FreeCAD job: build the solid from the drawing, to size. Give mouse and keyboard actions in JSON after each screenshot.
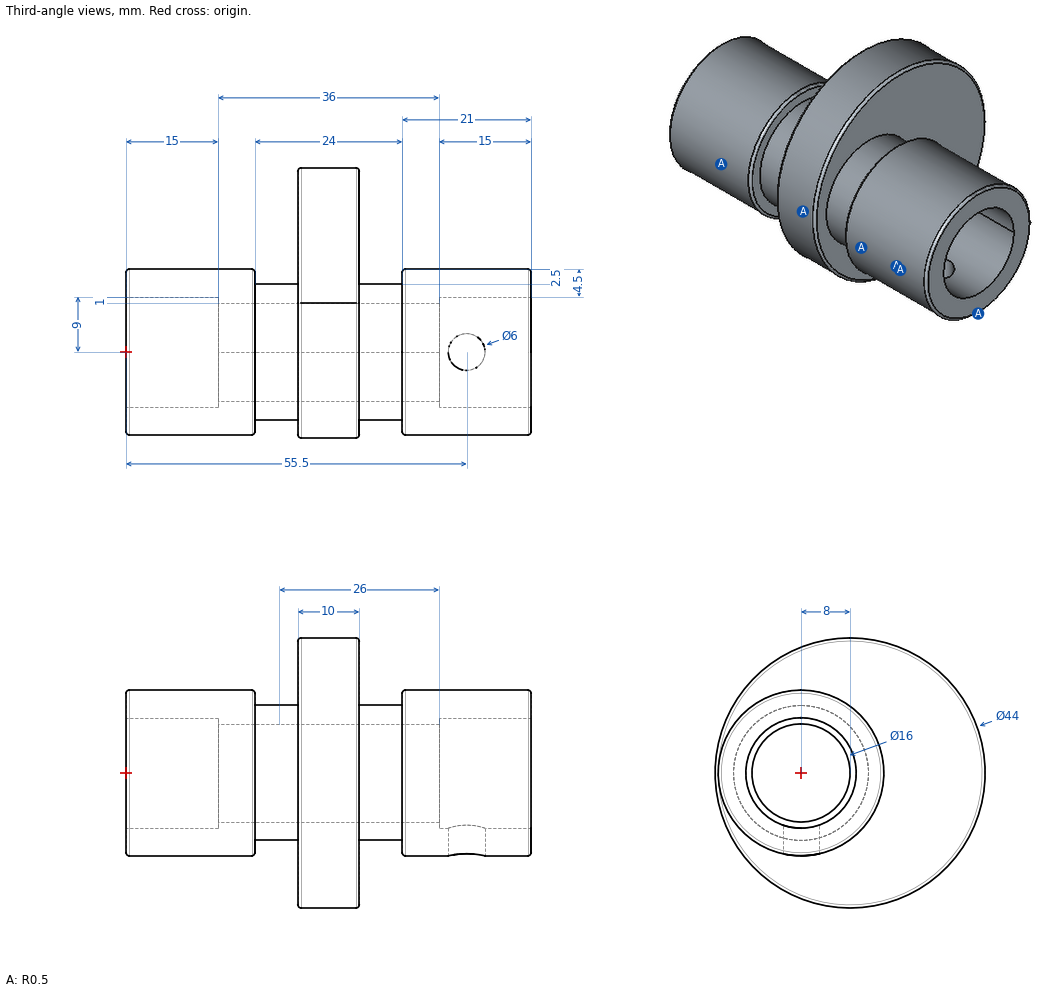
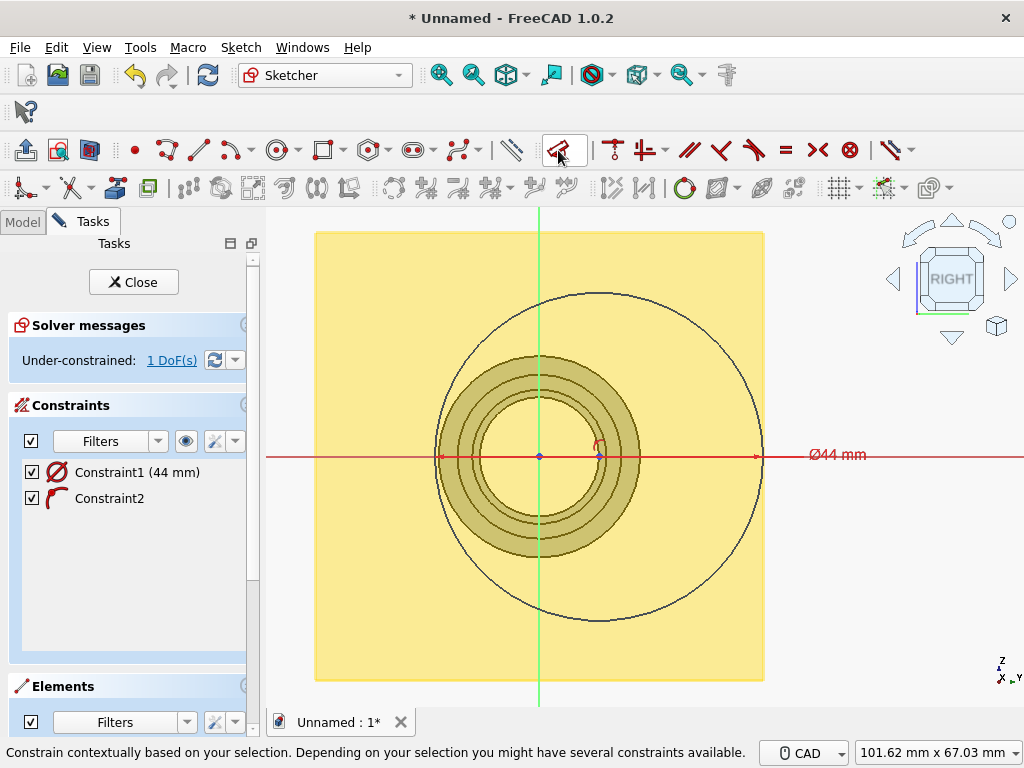
{"action": "left_click", "coordinate": [599, 457]}
{"action": "left_click", "coordinate": [569, 491]}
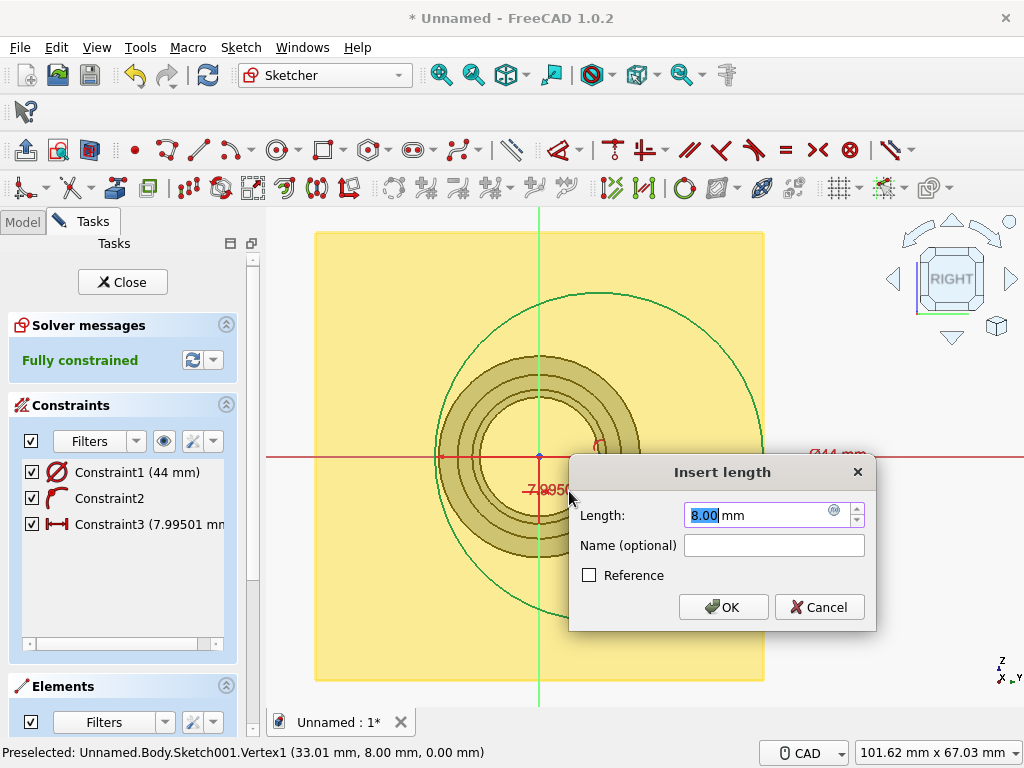
{"action": "type", "text": "8"}
{"action": "key", "text": "Return"}
{"action": "key", "text": "Escape"}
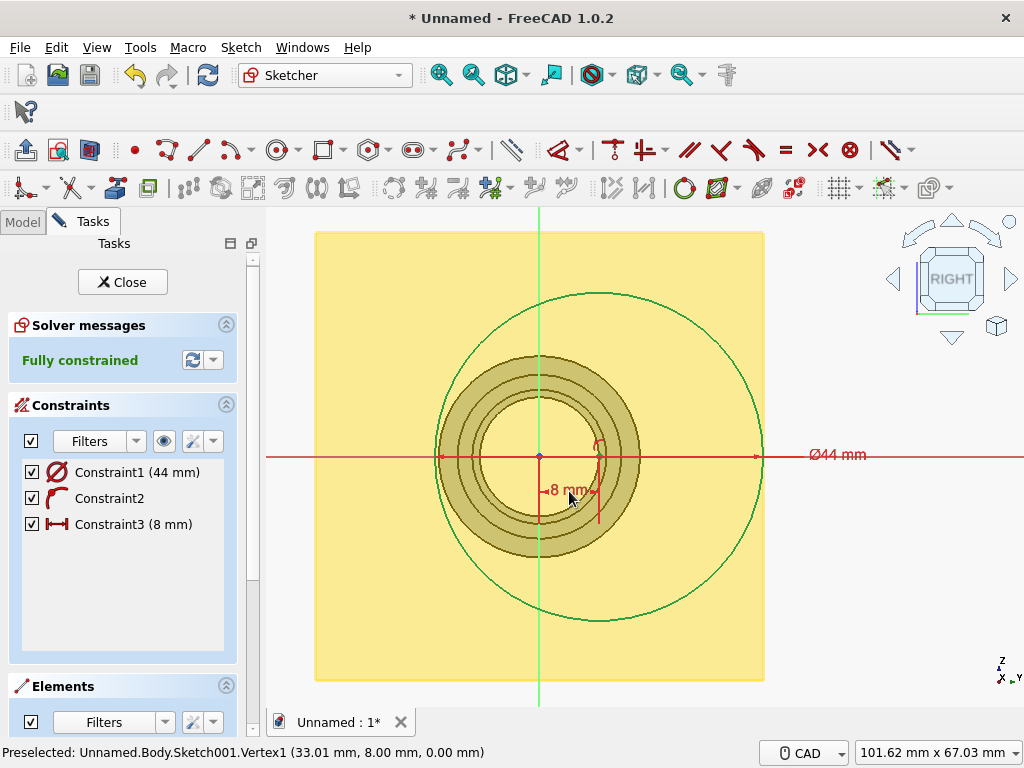
{"action": "left_click", "coordinate": [123, 282]}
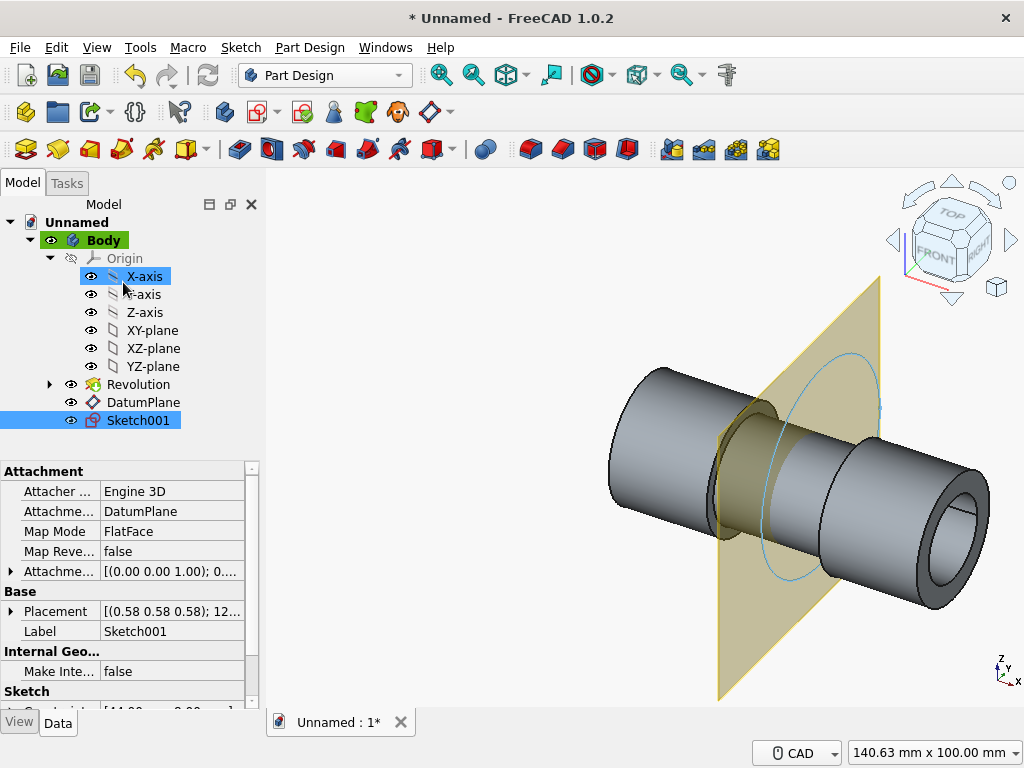
{"action": "left_click", "coordinate": [26, 150]}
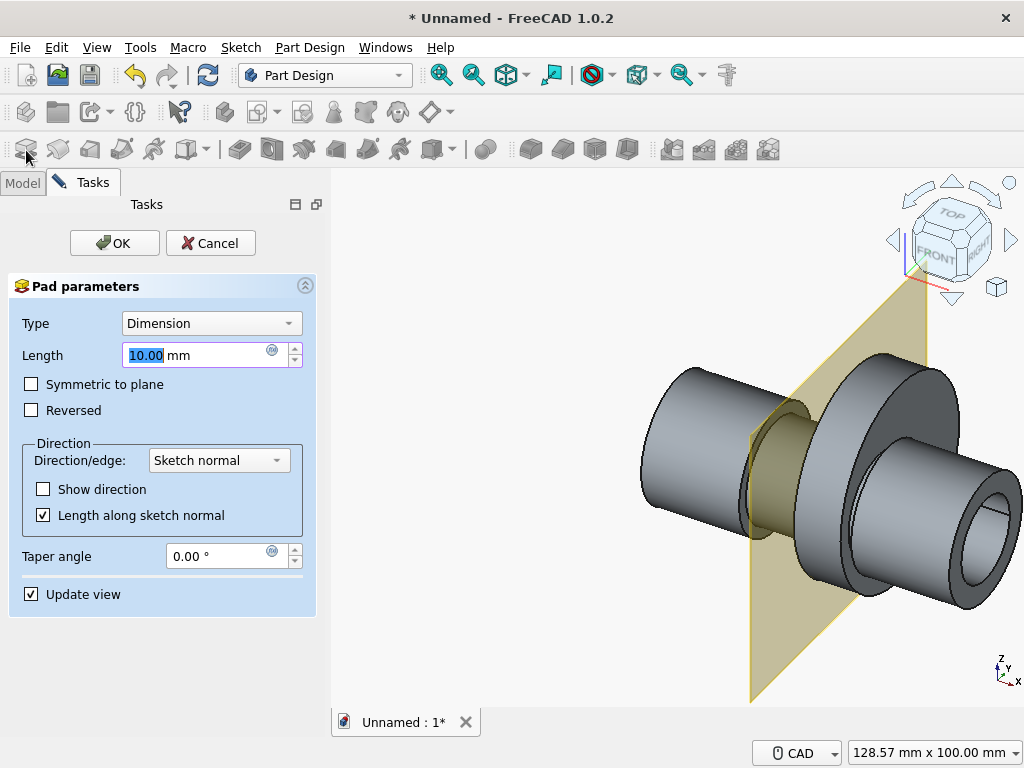
{"action": "type", "text": "10"}
{"action": "key", "text": "Tab"}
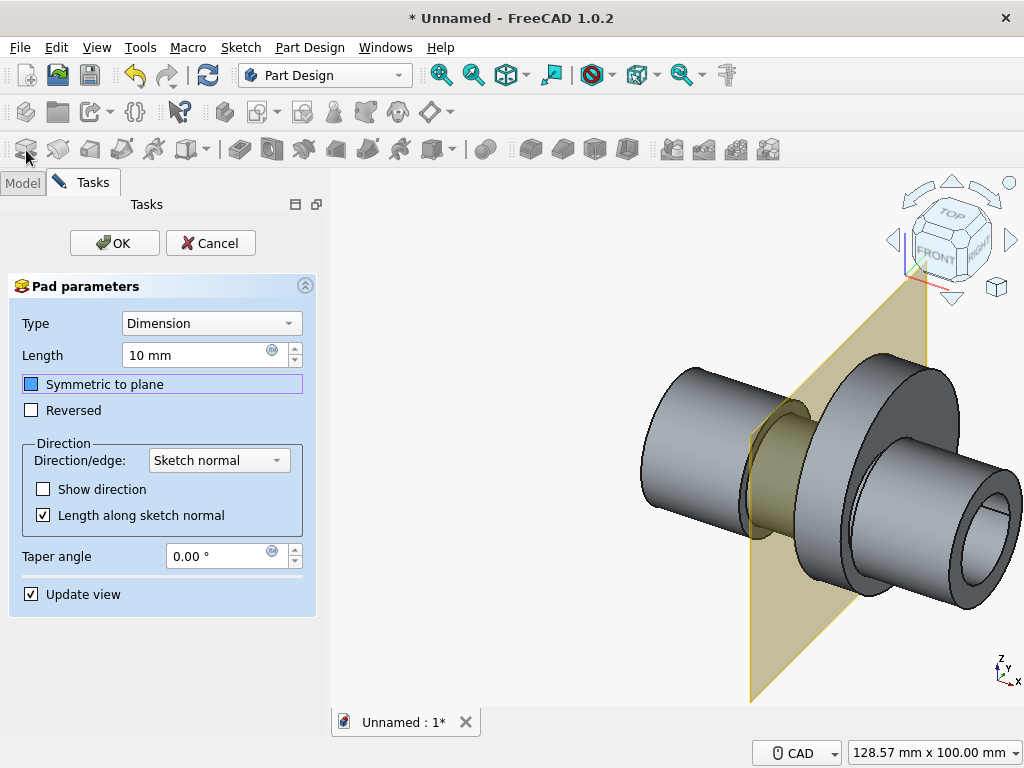
{"action": "left_click", "coordinate": [30, 384]}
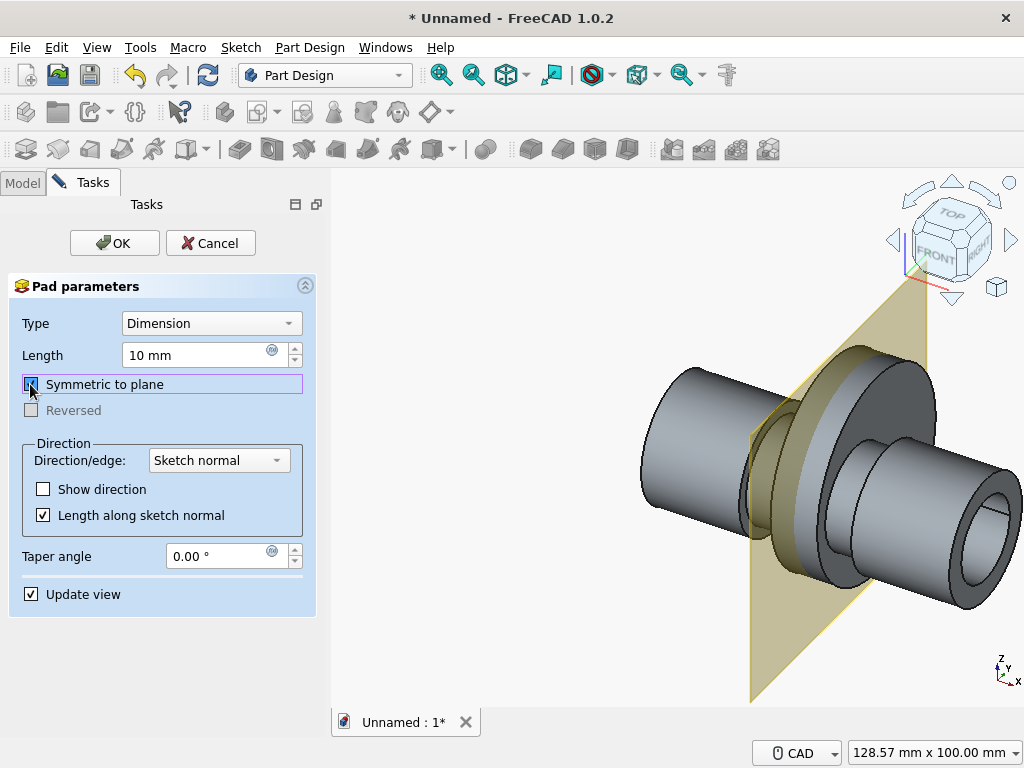
{"action": "left_click", "coordinate": [115, 243]}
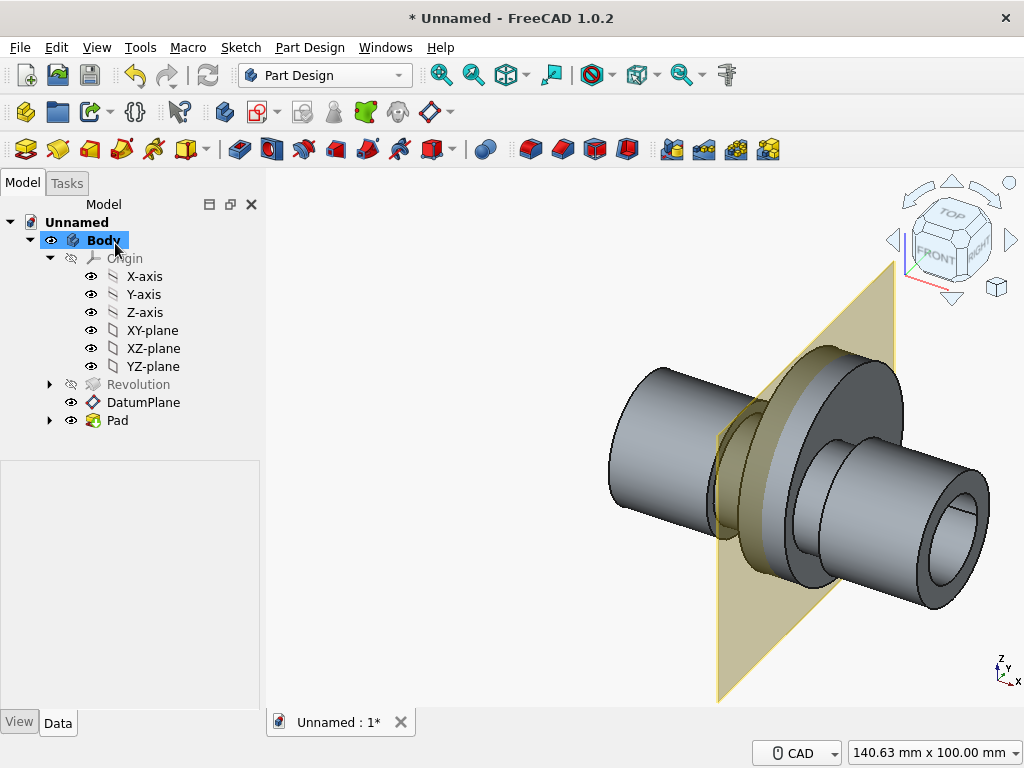
{"action": "left_click", "coordinate": [116, 402]}
{"action": "key", "text": "space"}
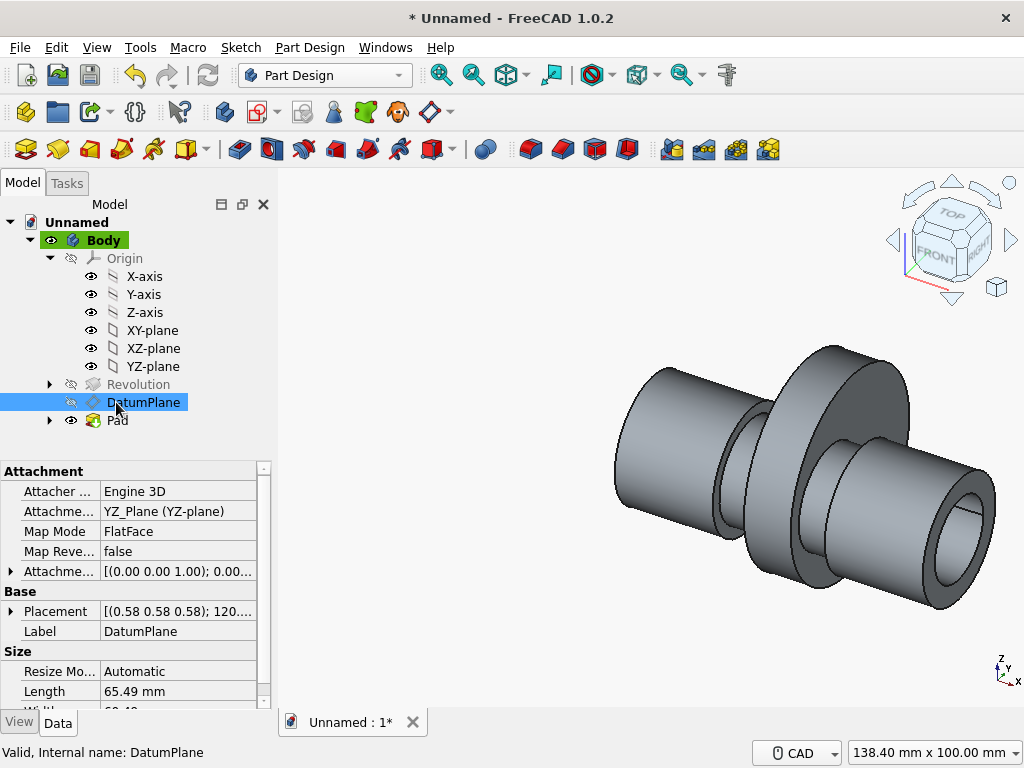
{"action": "left_click", "coordinate": [442, 76]}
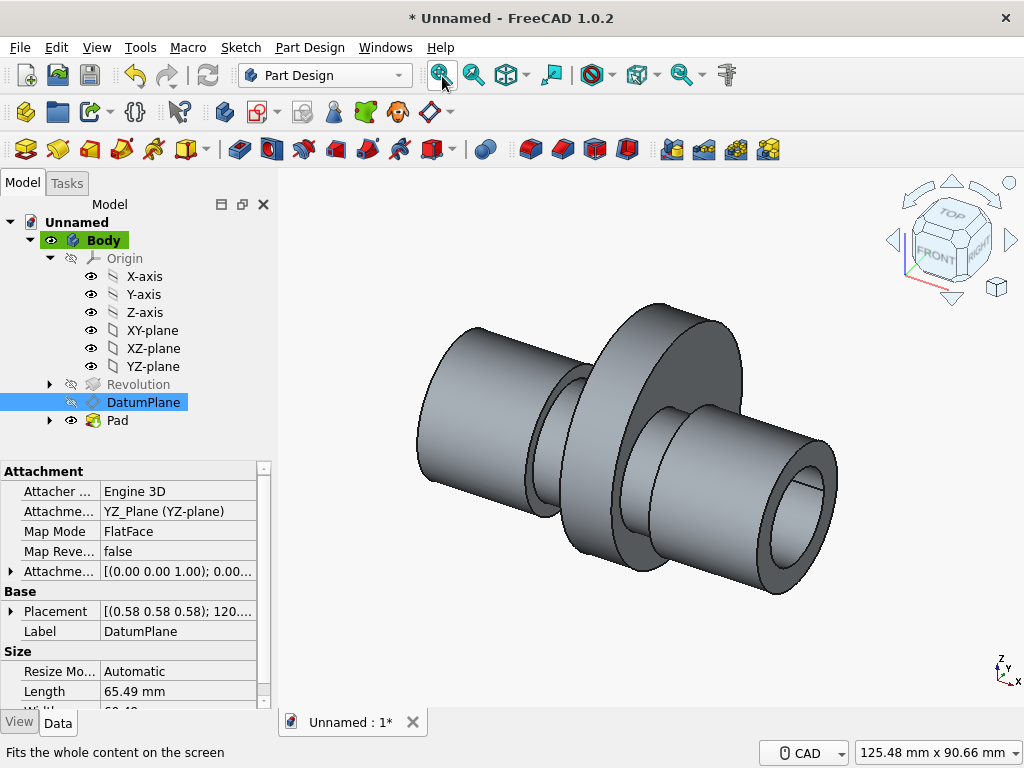
{"action": "left_click", "coordinate": [695, 365]}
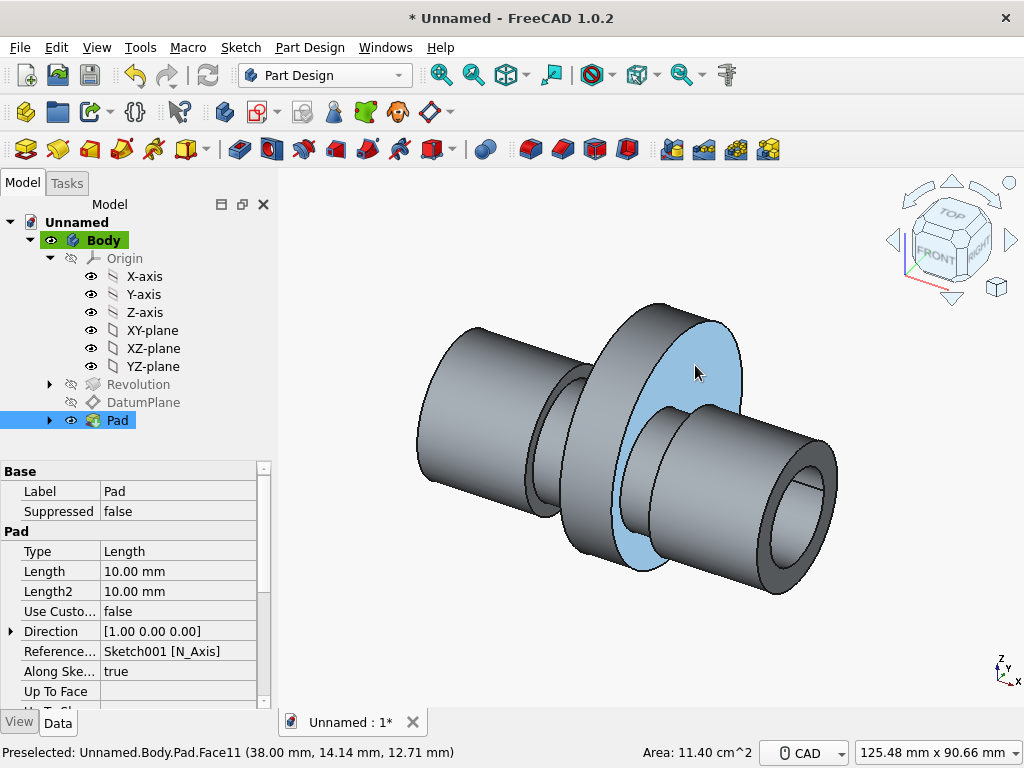
{"action": "left_click", "coordinate": [258, 112]}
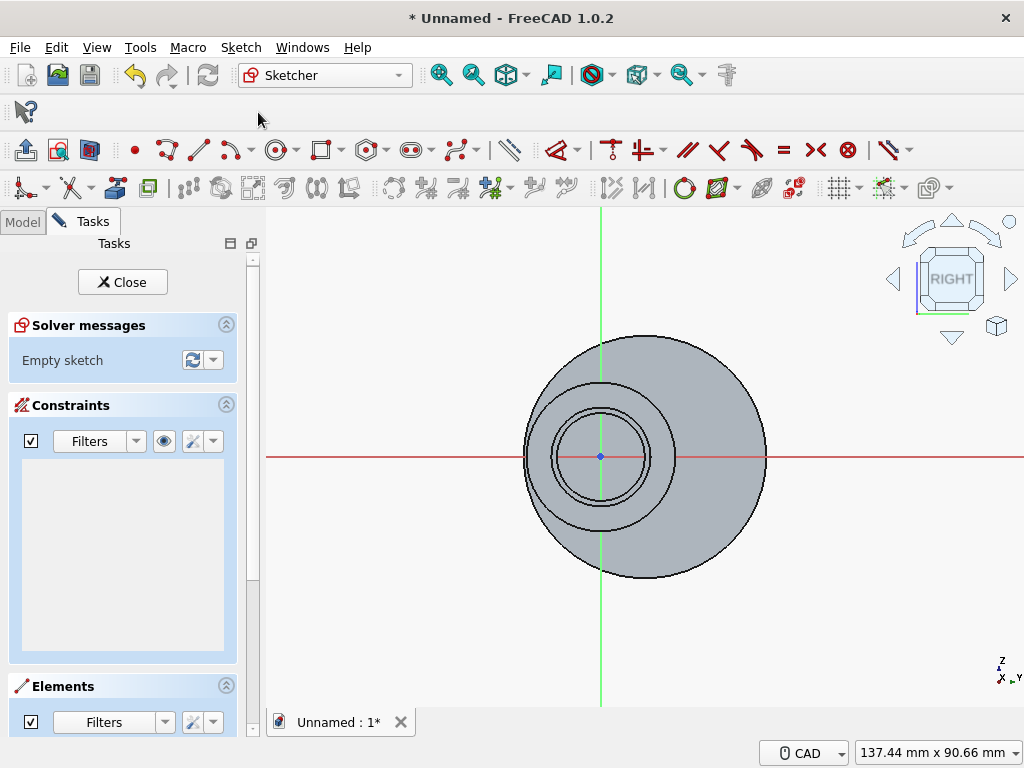
{"action": "scroll", "coordinate": [611, 457], "scroll_direction": "up", "scroll_amount": 6}